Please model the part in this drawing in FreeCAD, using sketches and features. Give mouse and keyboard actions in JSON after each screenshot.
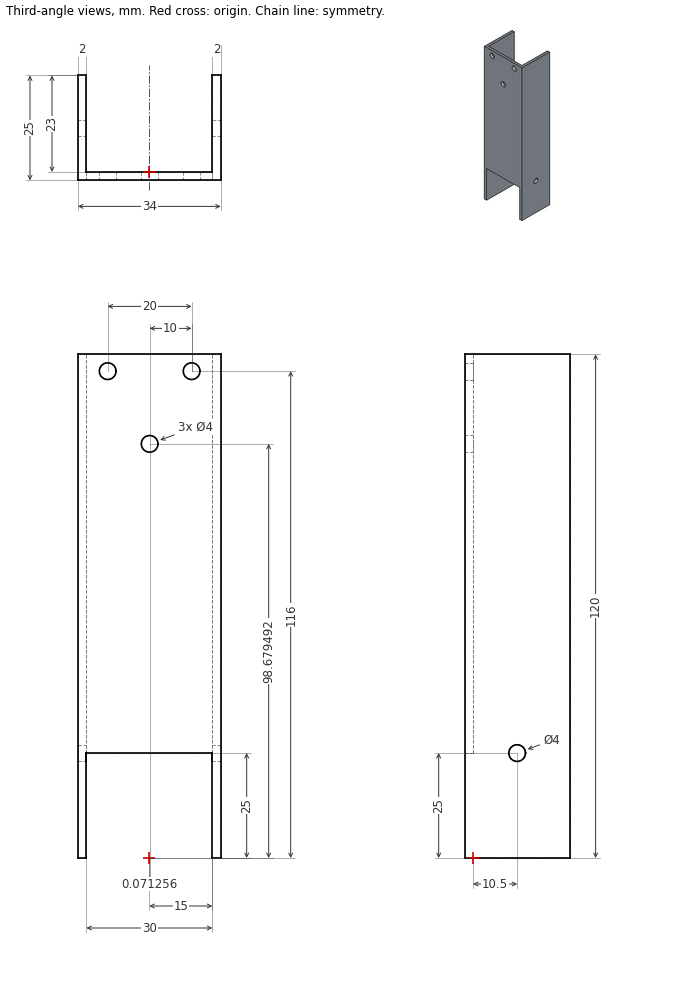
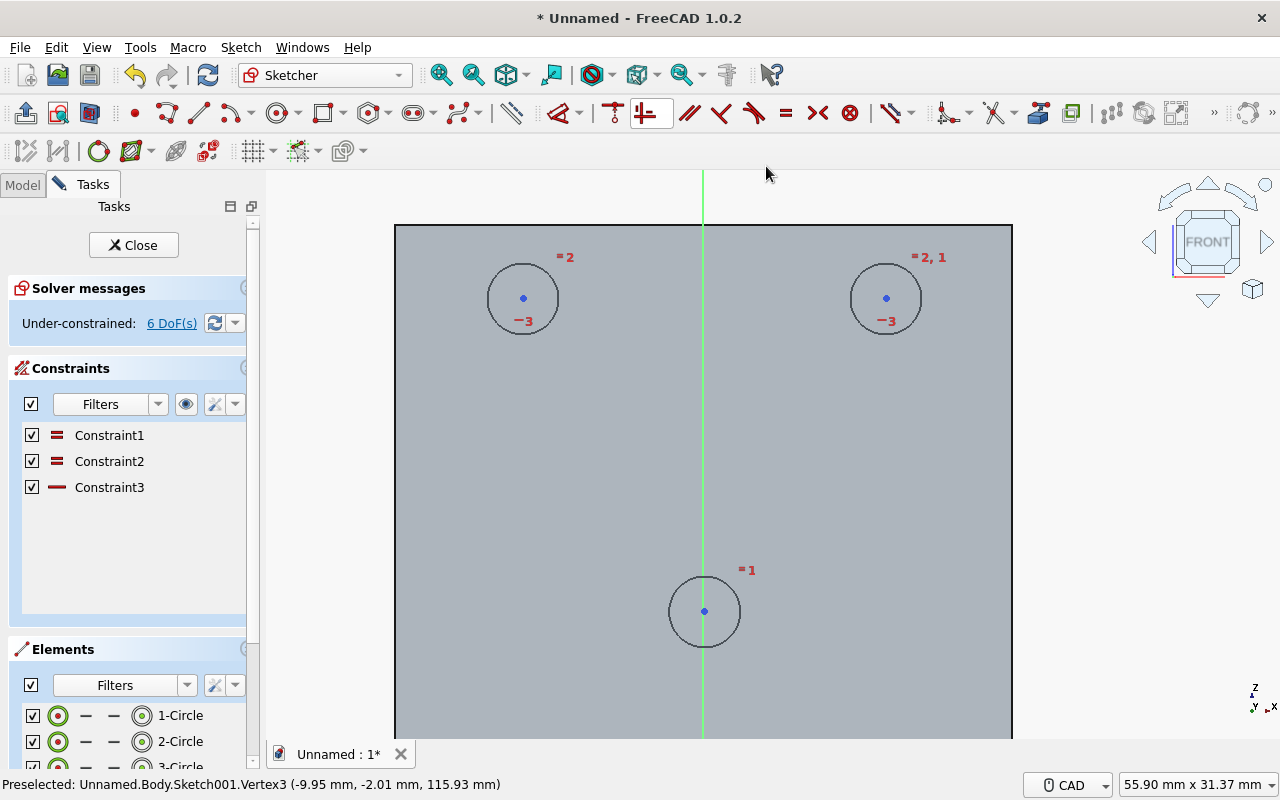
{"action": "left_click", "coordinate": [558, 114]}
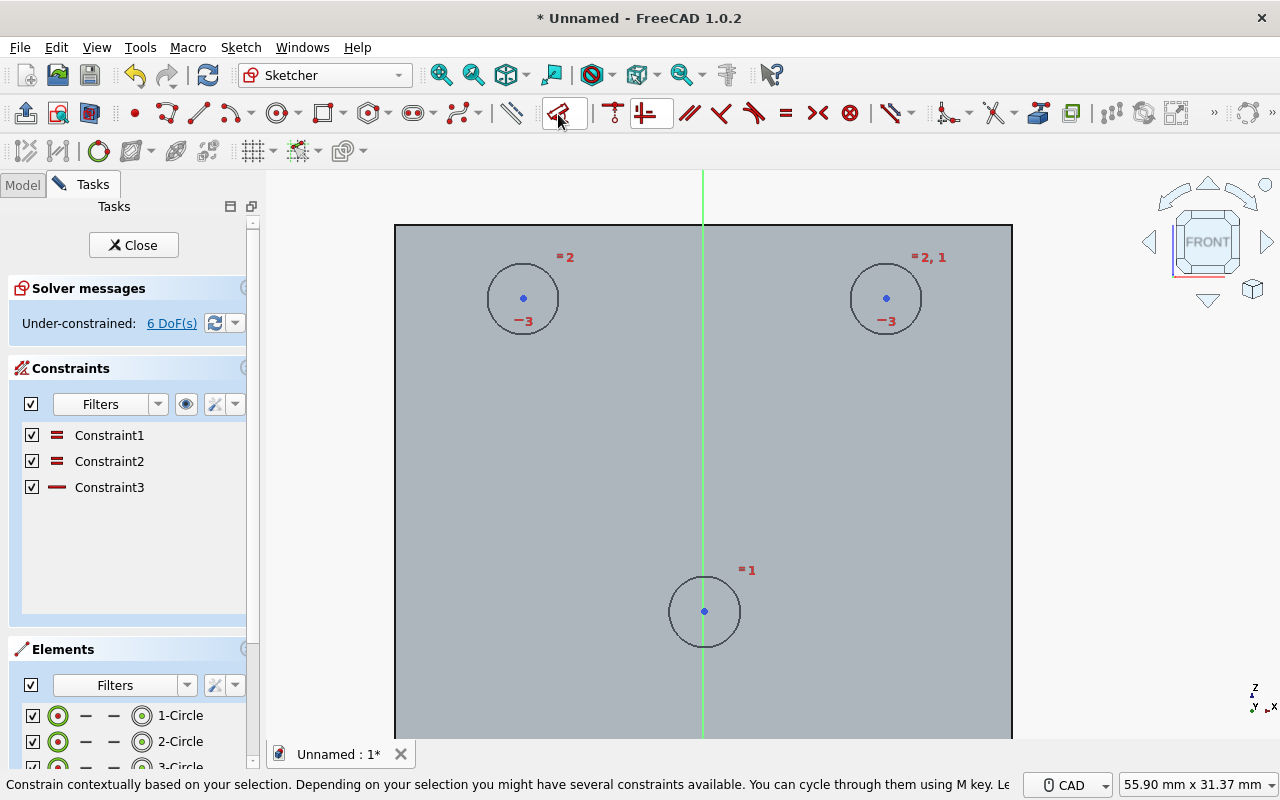
{"action": "left_click", "coordinate": [730, 587]}
{"action": "left_click", "coordinate": [753, 565]}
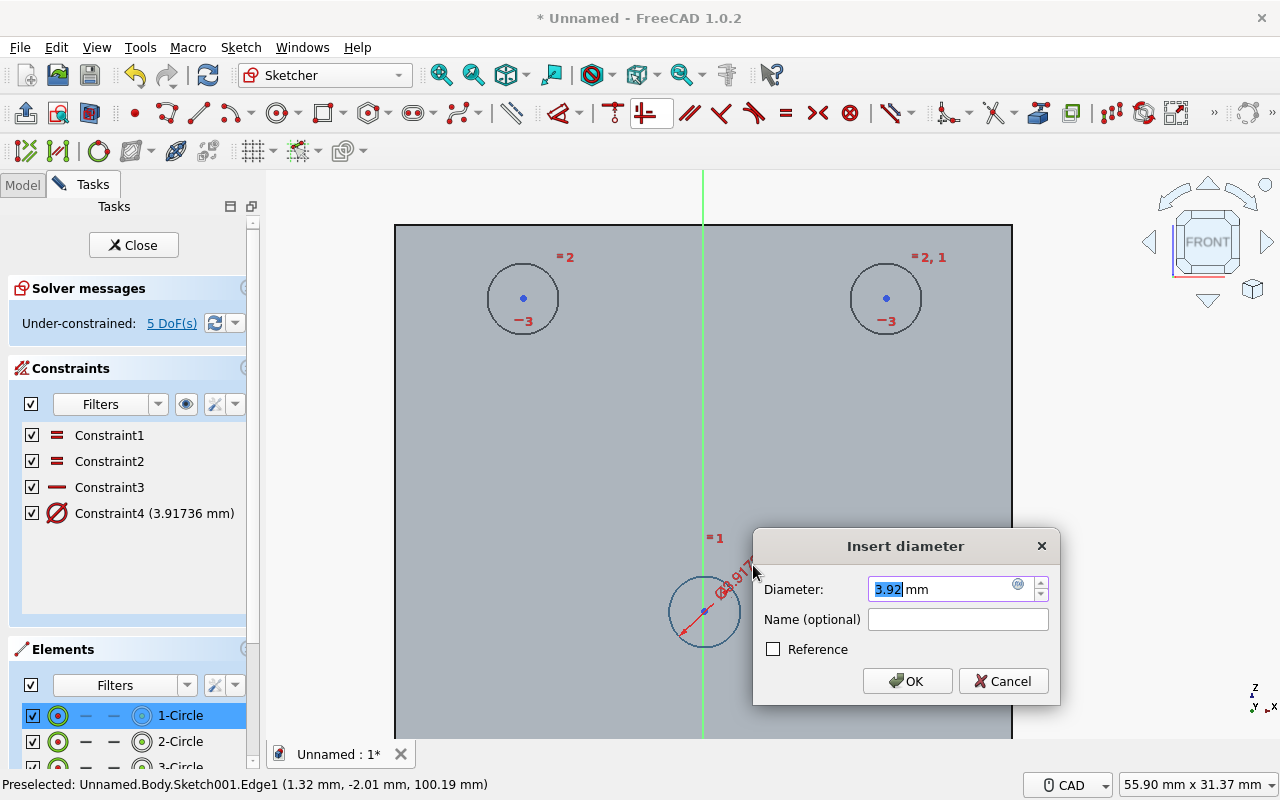
{"action": "type", "text": "4"}
{"action": "key", "text": "Return"}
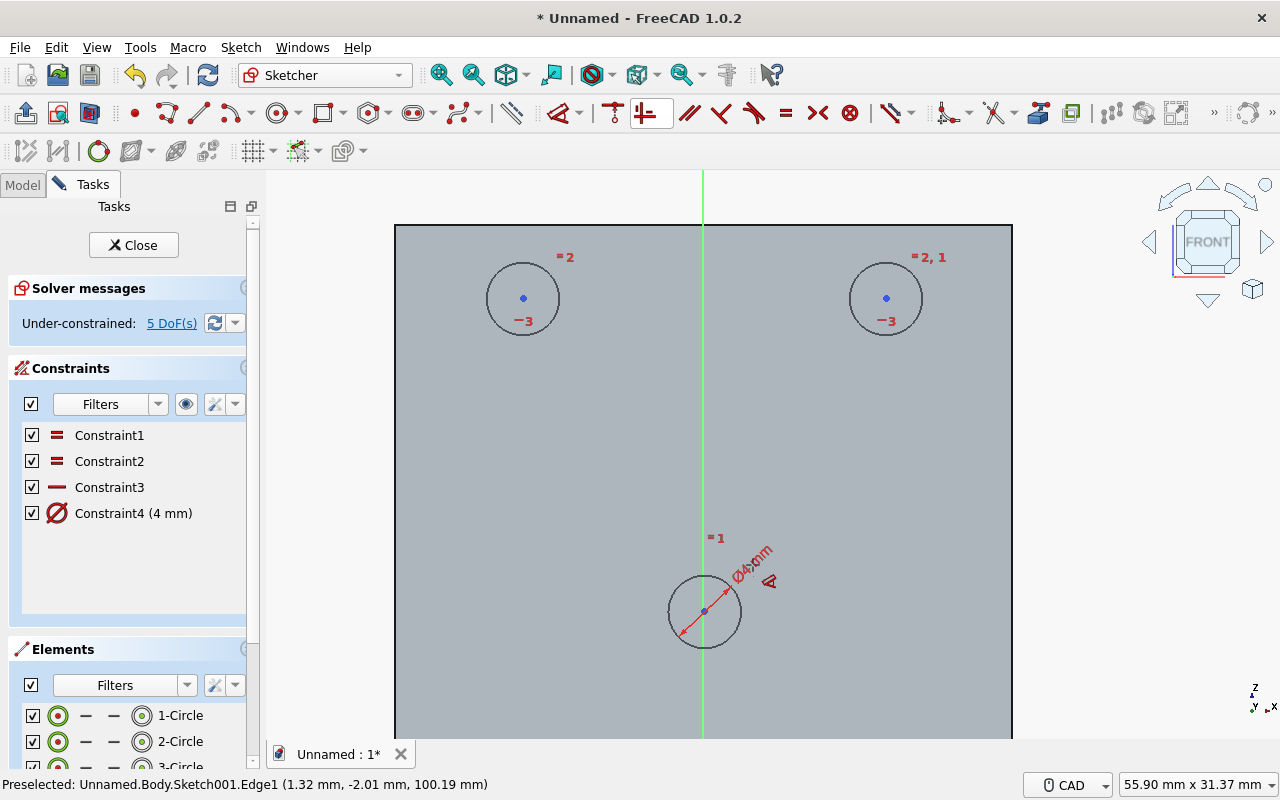
{"action": "left_click", "coordinate": [886, 299]}
{"action": "left_click", "coordinate": [920, 505]}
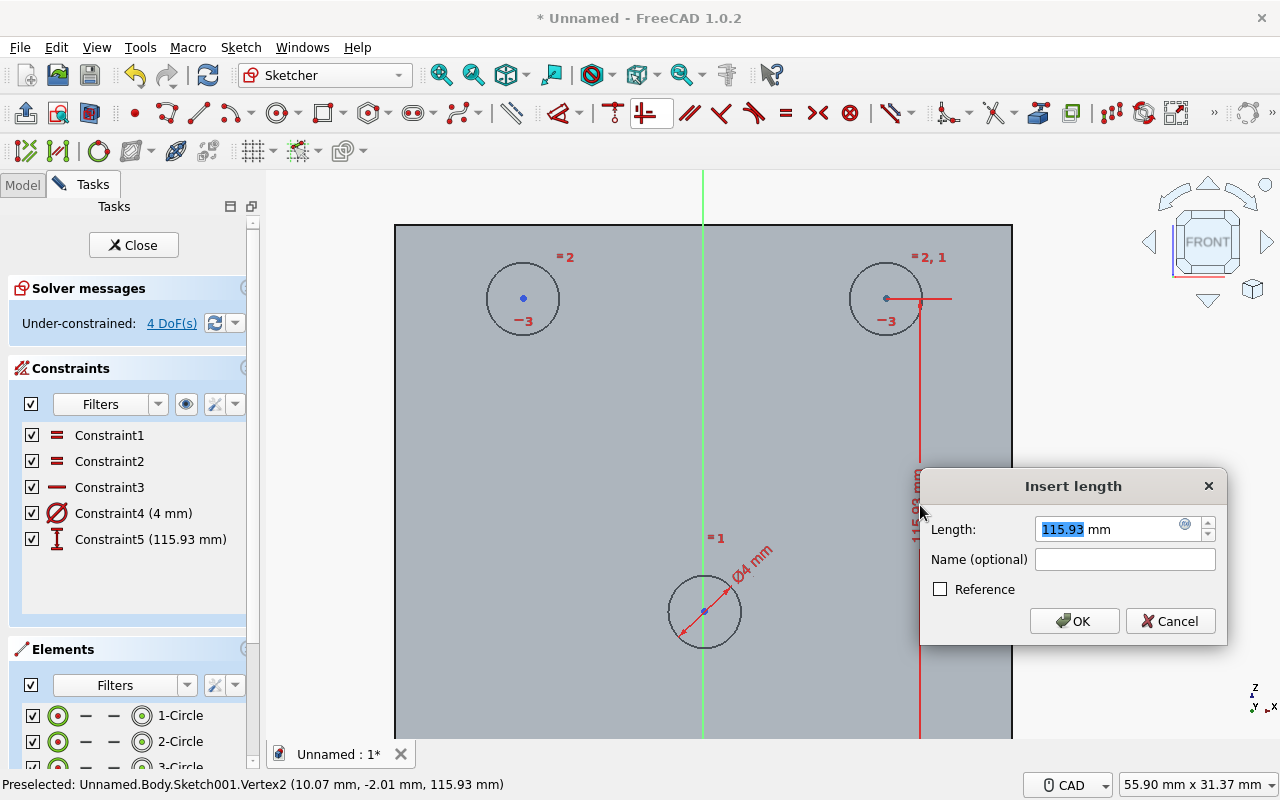
{"action": "type", "text": "116"}
{"action": "key", "text": "Return"}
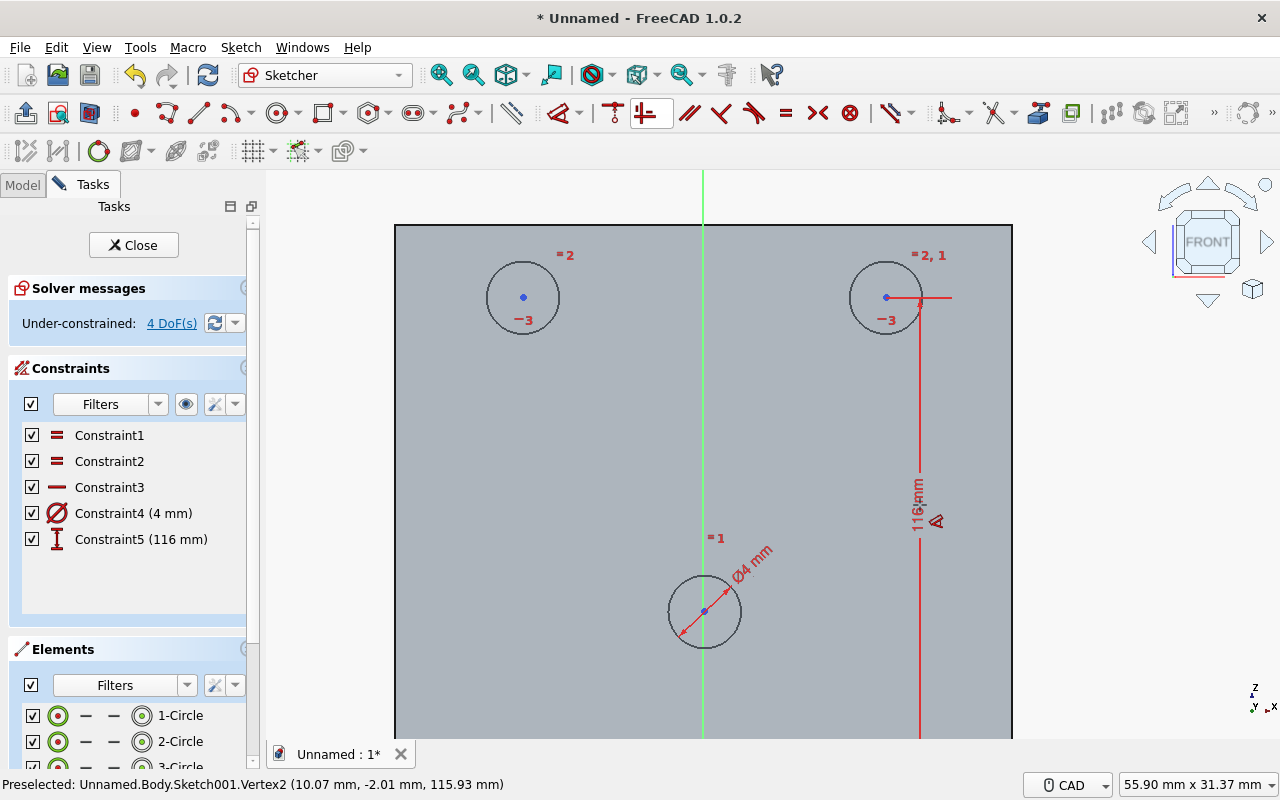
{"action": "left_click", "coordinate": [705, 612]}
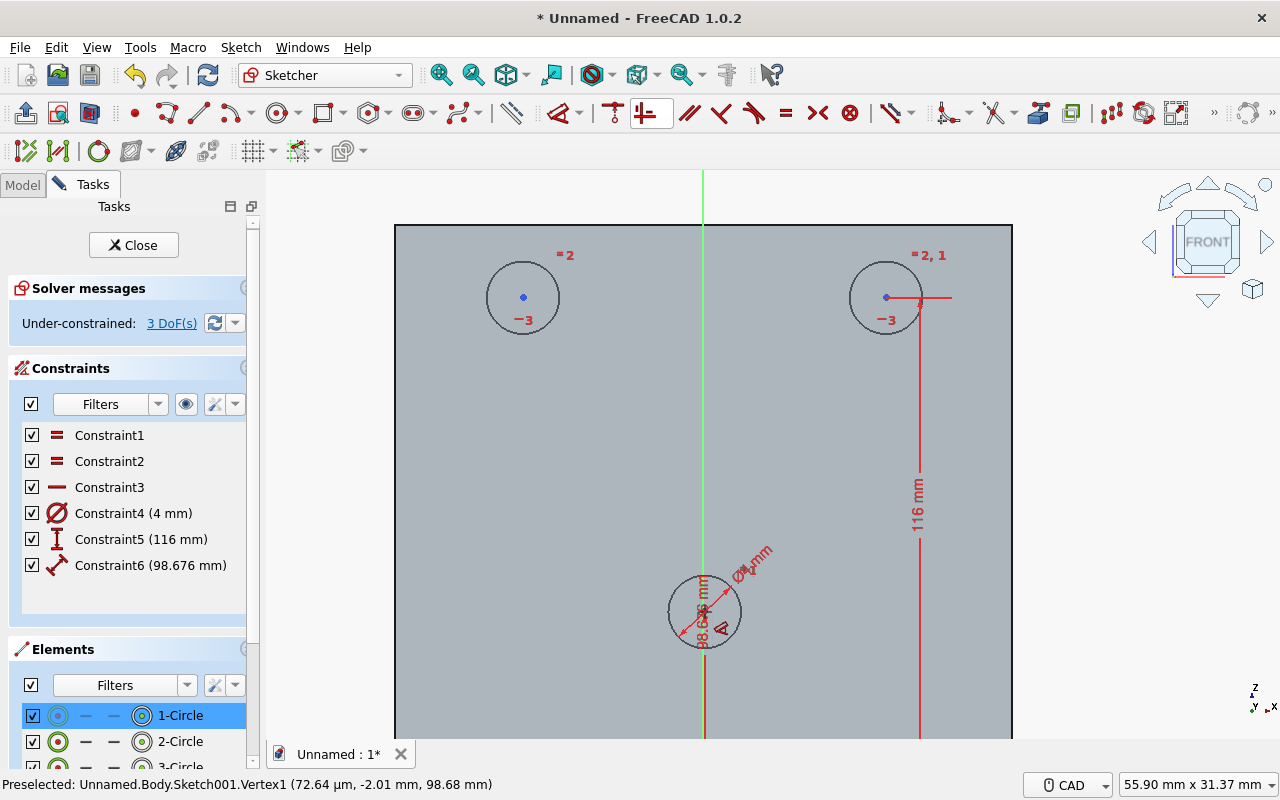
{"action": "left_click", "coordinate": [886, 298]}
{"action": "left_click", "coordinate": [795, 646]}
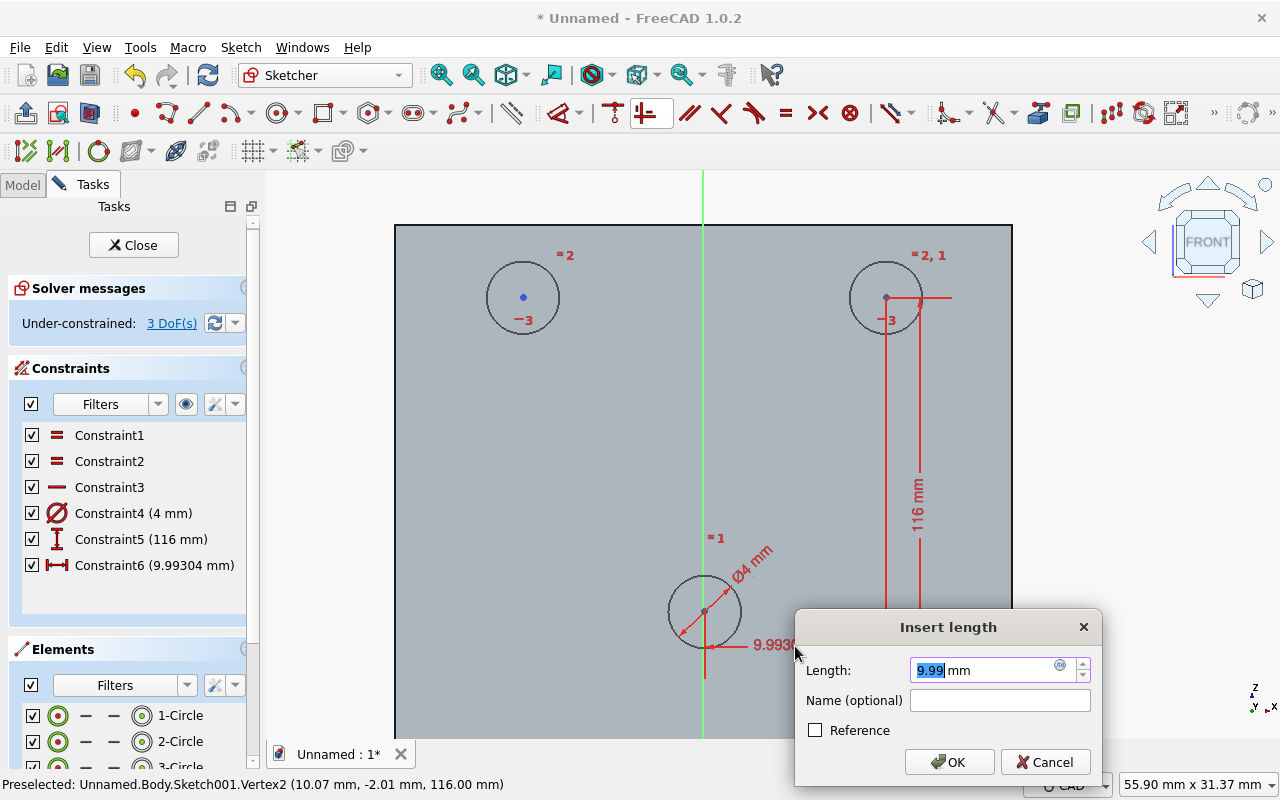
{"action": "type", "text": "10"}
{"action": "key", "text": "Return"}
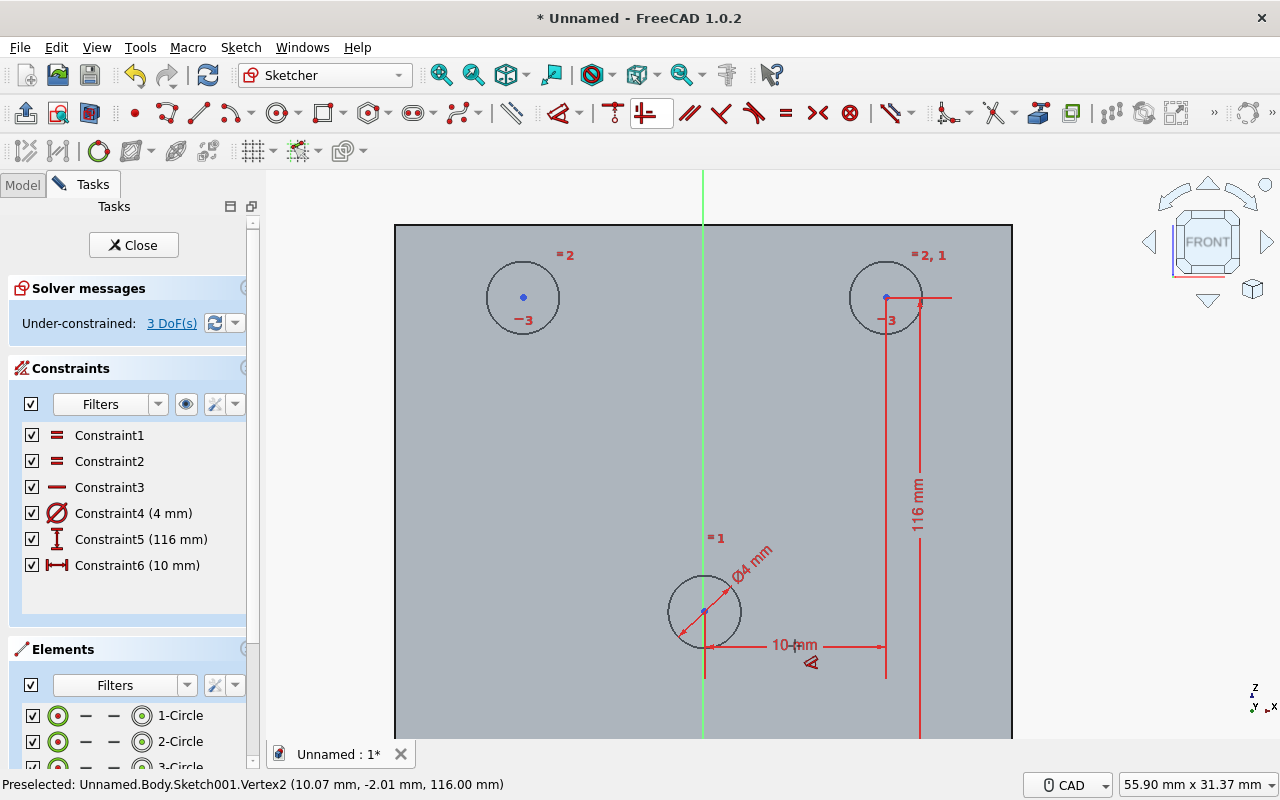
{"action": "left_click", "coordinate": [886, 298]}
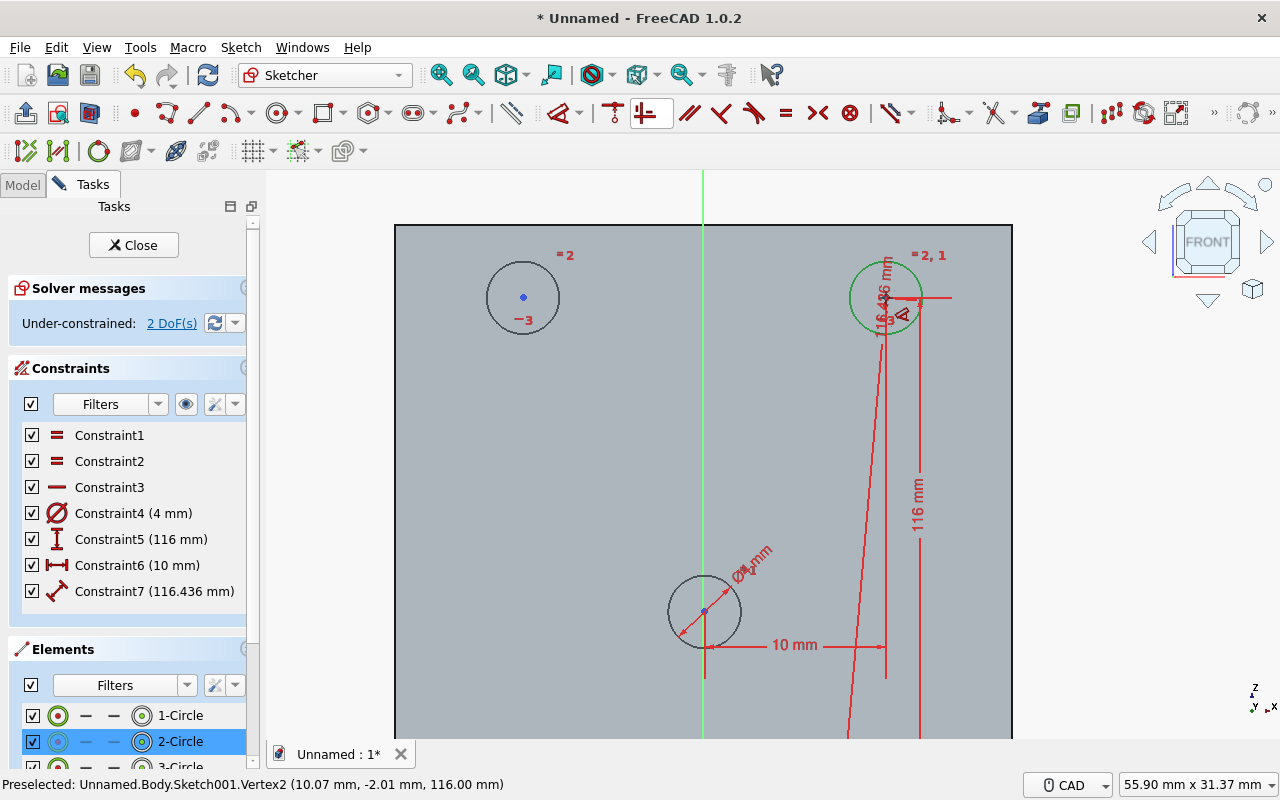
{"action": "left_click", "coordinate": [523, 298]}
{"action": "left_click", "coordinate": [621, 264]}